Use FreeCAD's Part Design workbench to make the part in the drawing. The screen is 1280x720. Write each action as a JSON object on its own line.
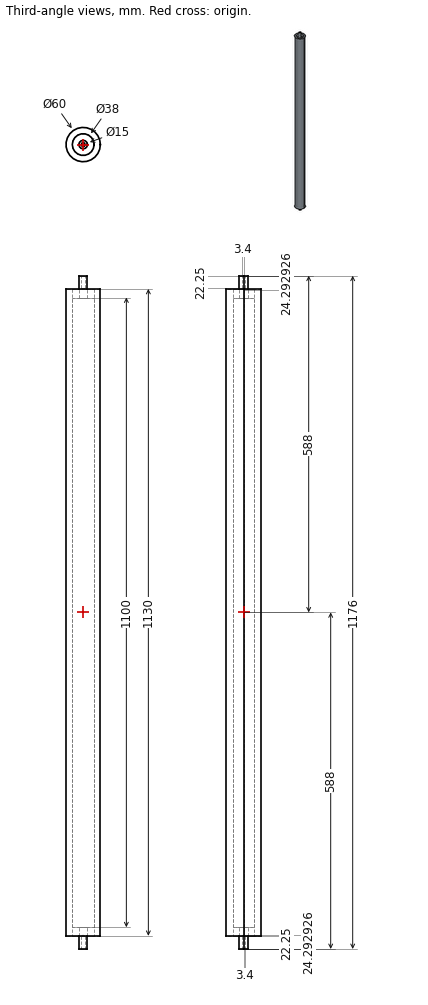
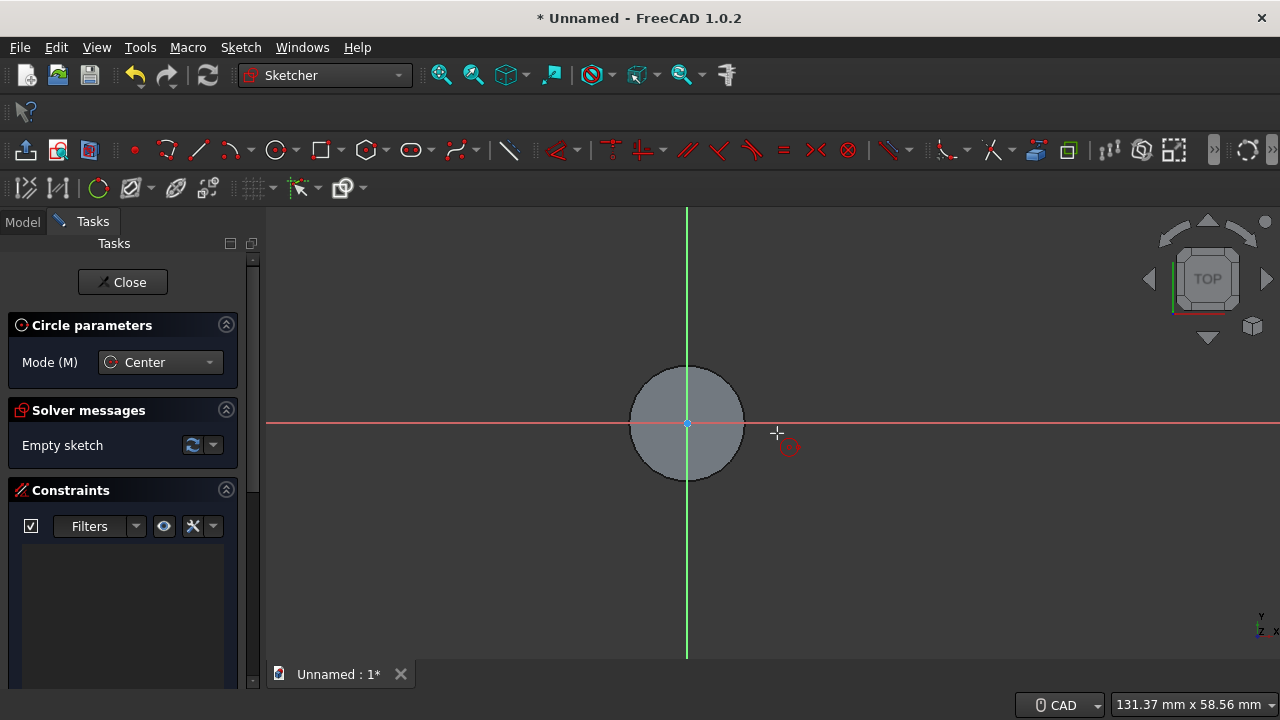
{"action": "left_click", "coordinate": [687, 423]}
{"action": "left_click", "coordinate": [791, 320]}
{"action": "key", "text": "Escape"}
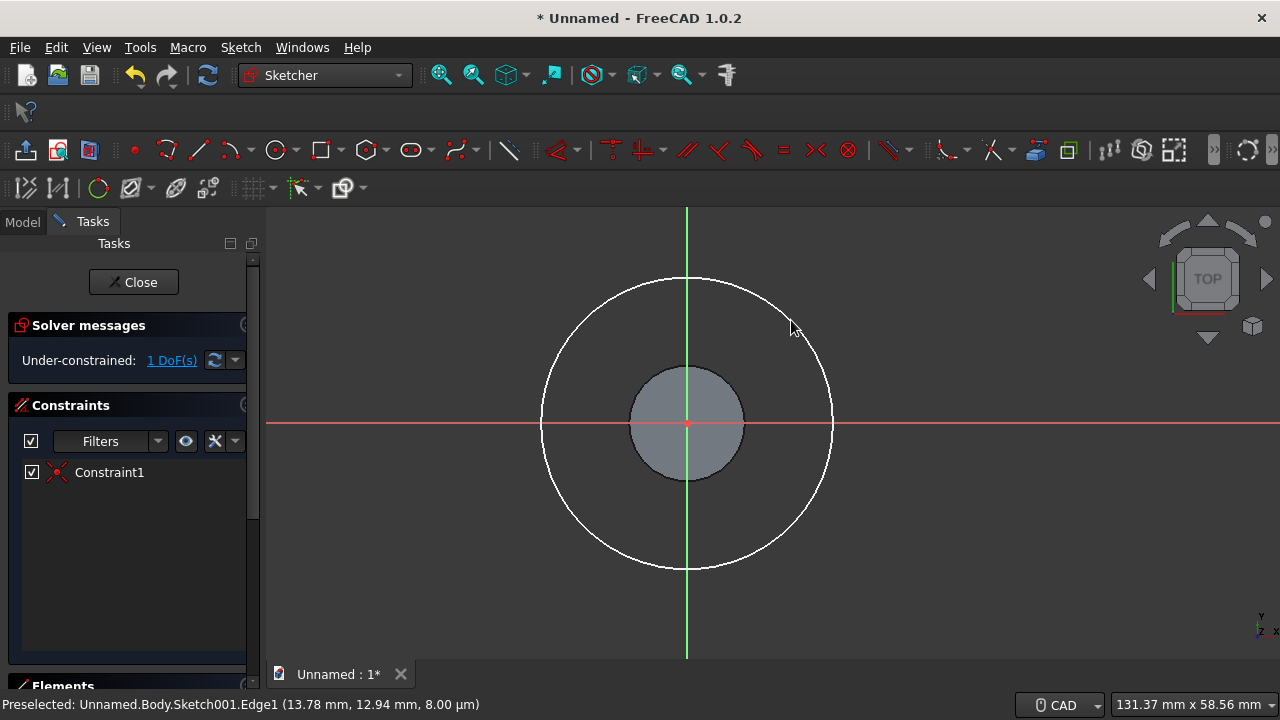
{"action": "left_click", "coordinate": [556, 150]}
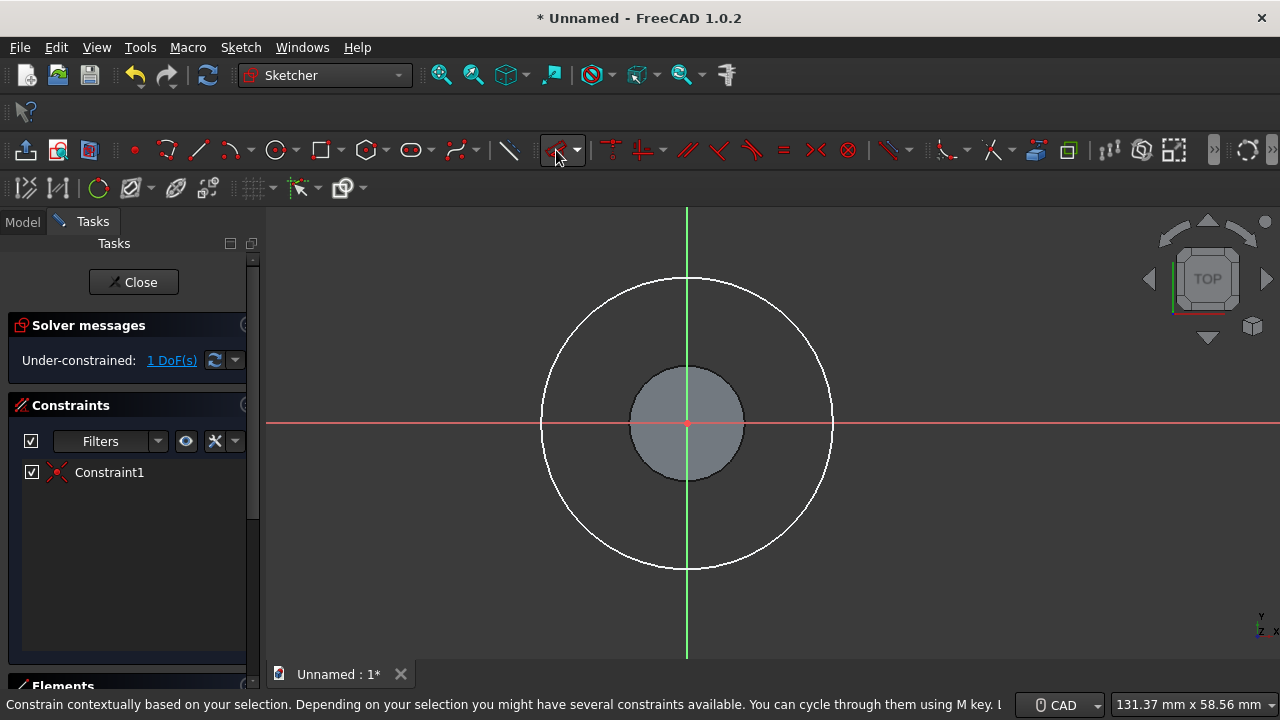
{"action": "left_click", "coordinate": [790, 320]}
{"action": "left_click", "coordinate": [813, 297]}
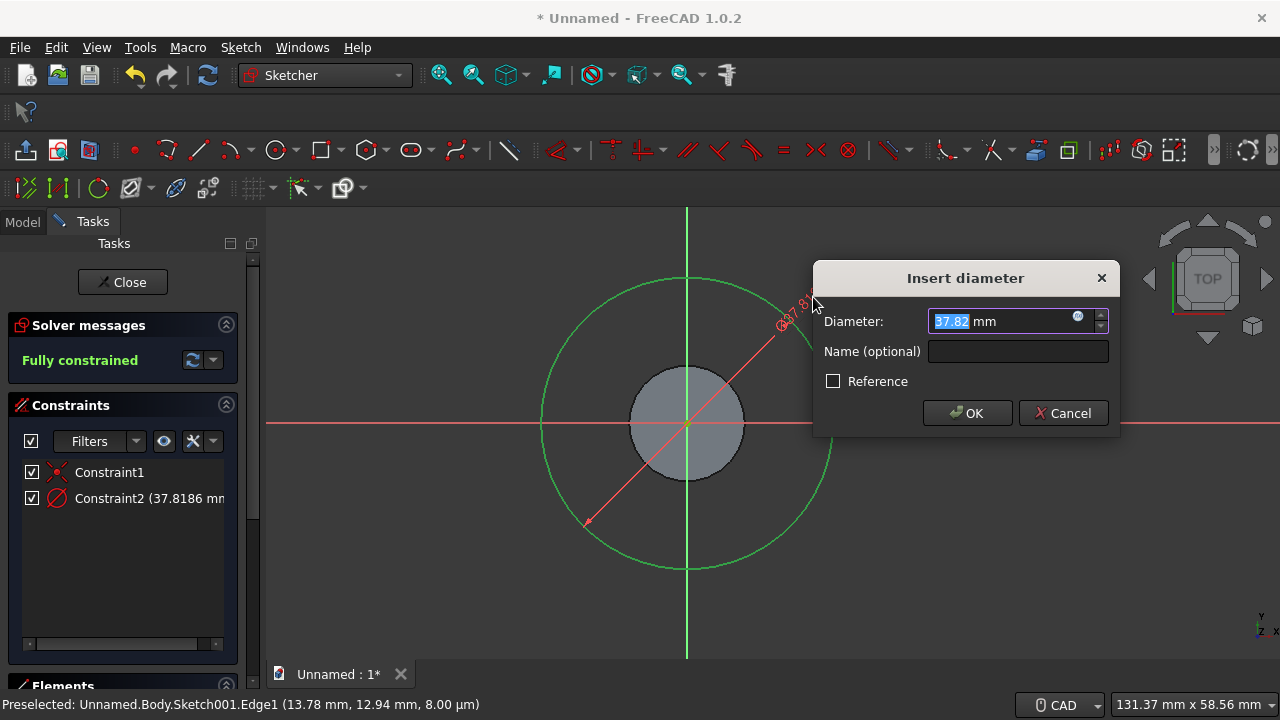
{"action": "type", "text": "38"}
{"action": "key", "text": "Return"}
{"action": "key", "text": "Escape"}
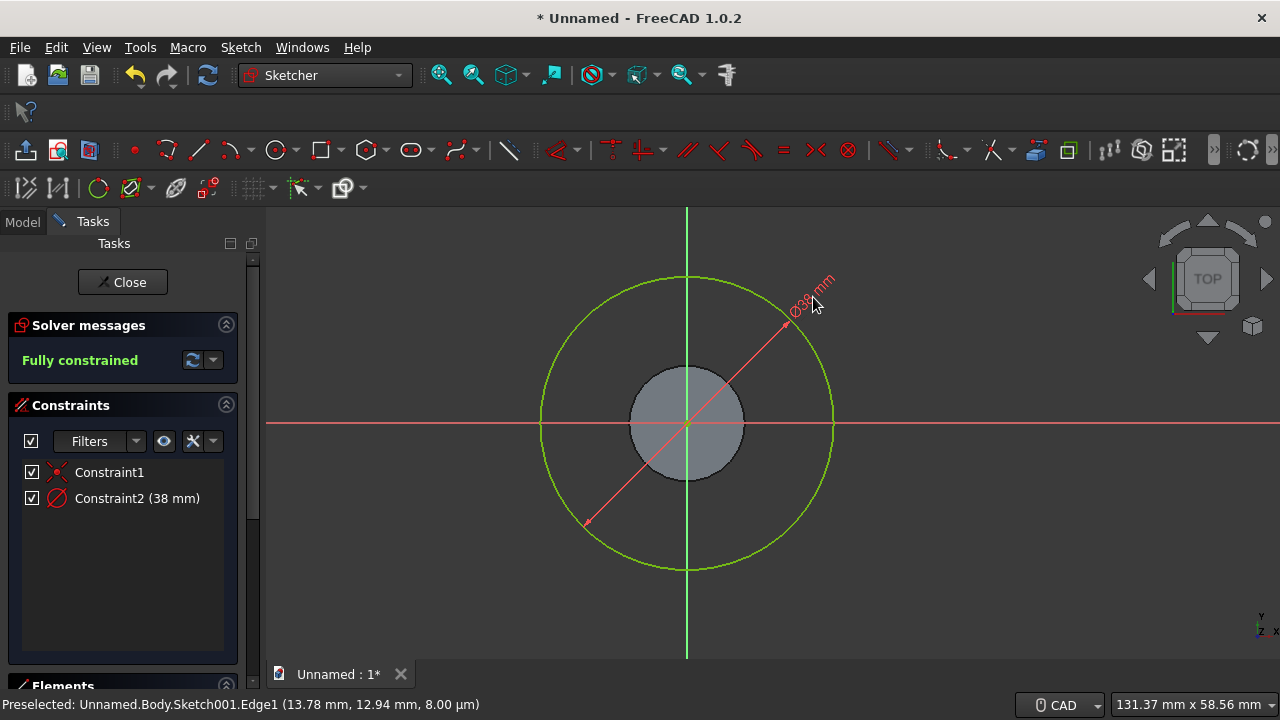
{"action": "left_click", "coordinate": [123, 282]}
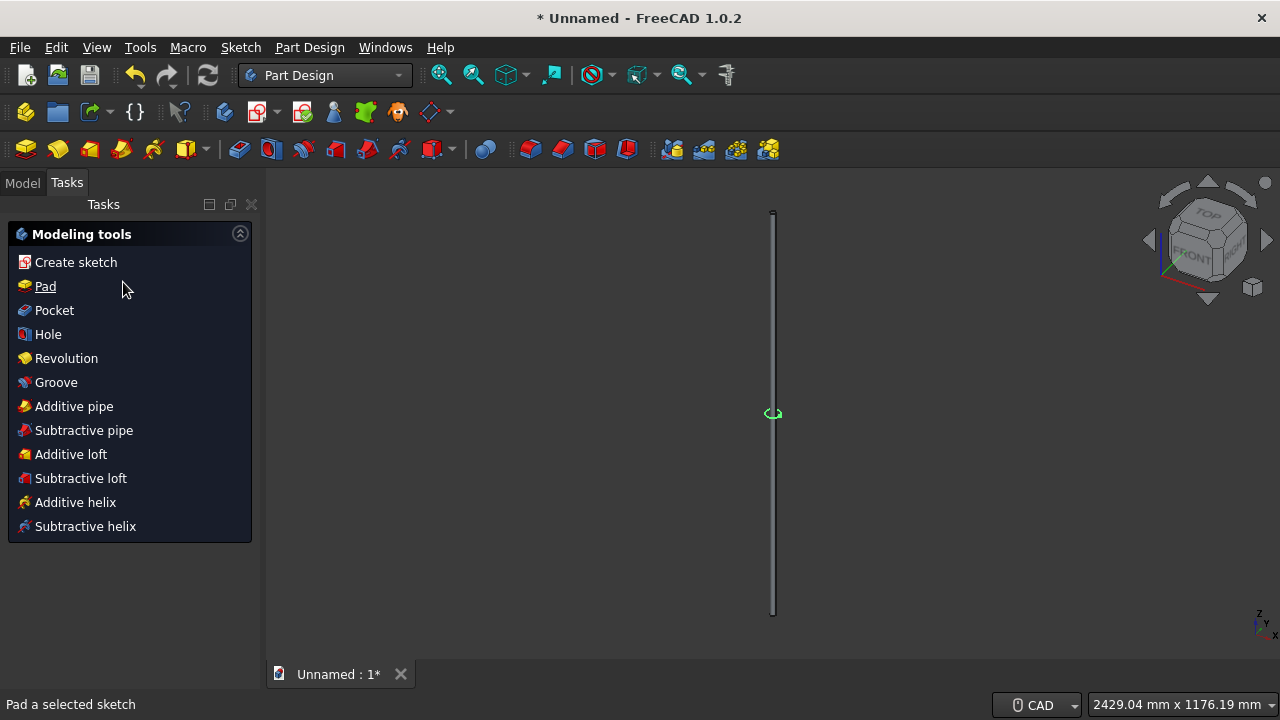
{"action": "left_click", "coordinate": [26, 150]}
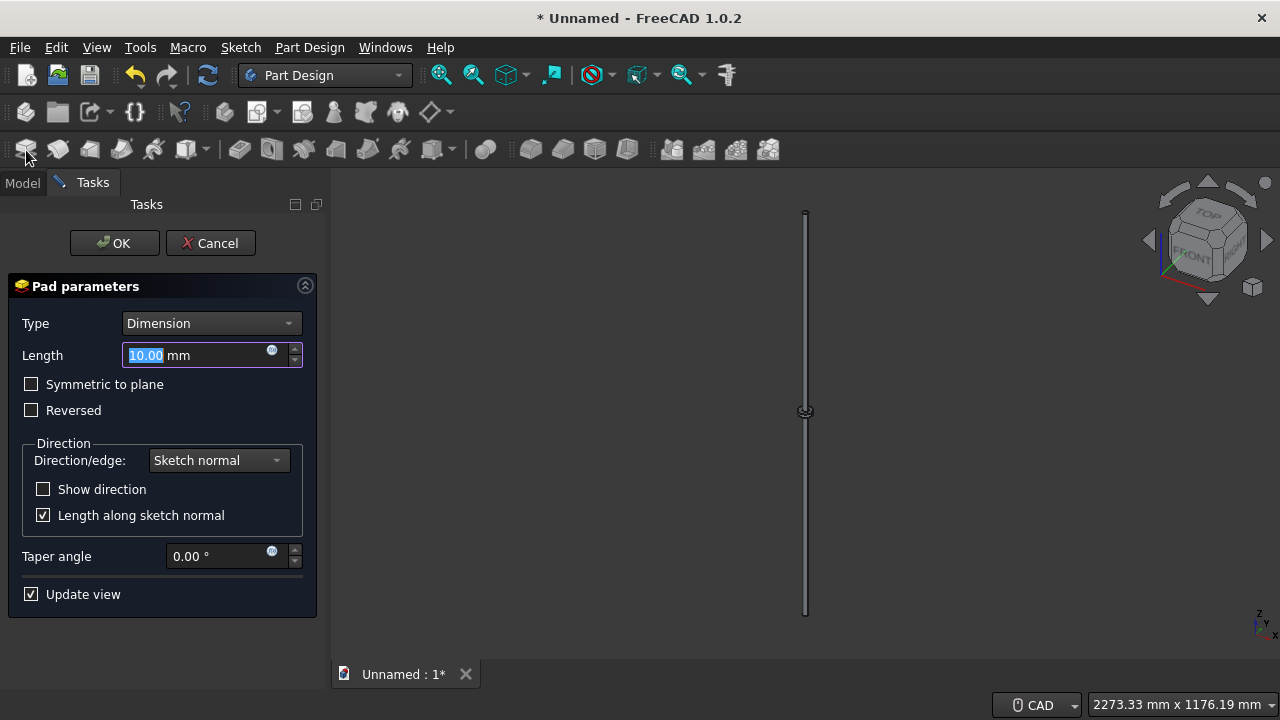
{"action": "type", "text": "1100"}
{"action": "key", "text": "Tab"}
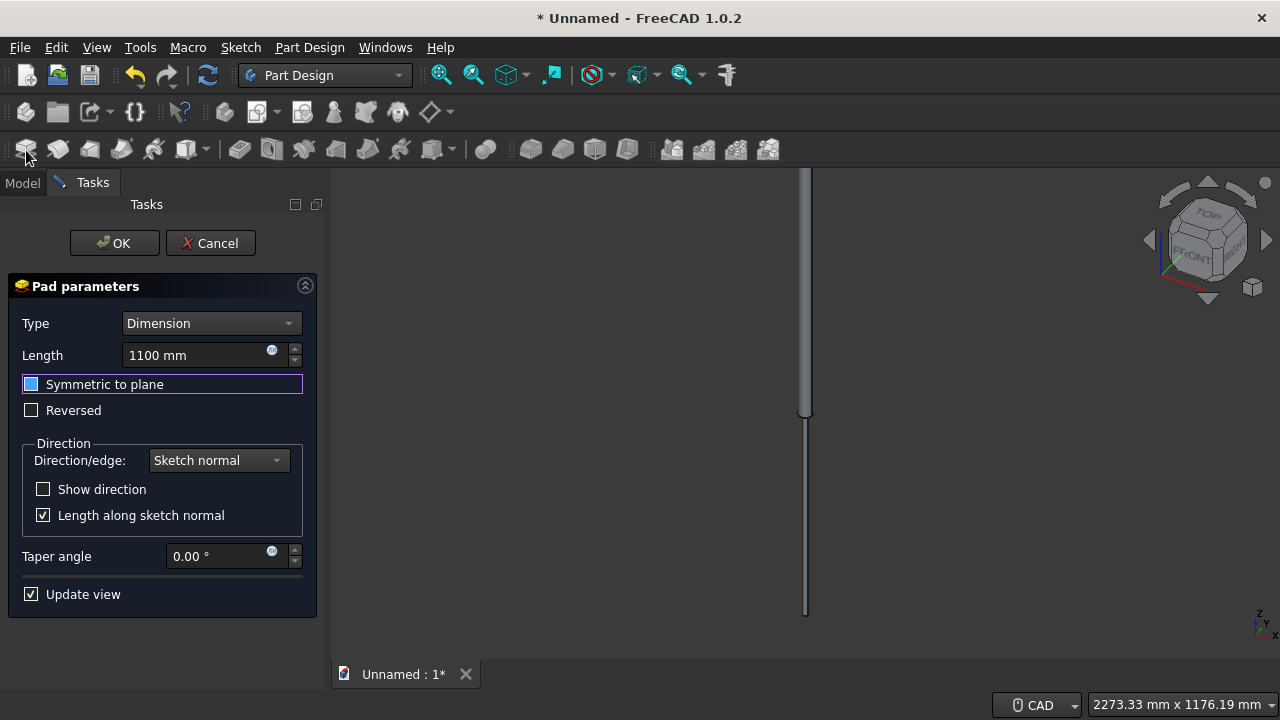
{"action": "left_click", "coordinate": [30, 384]}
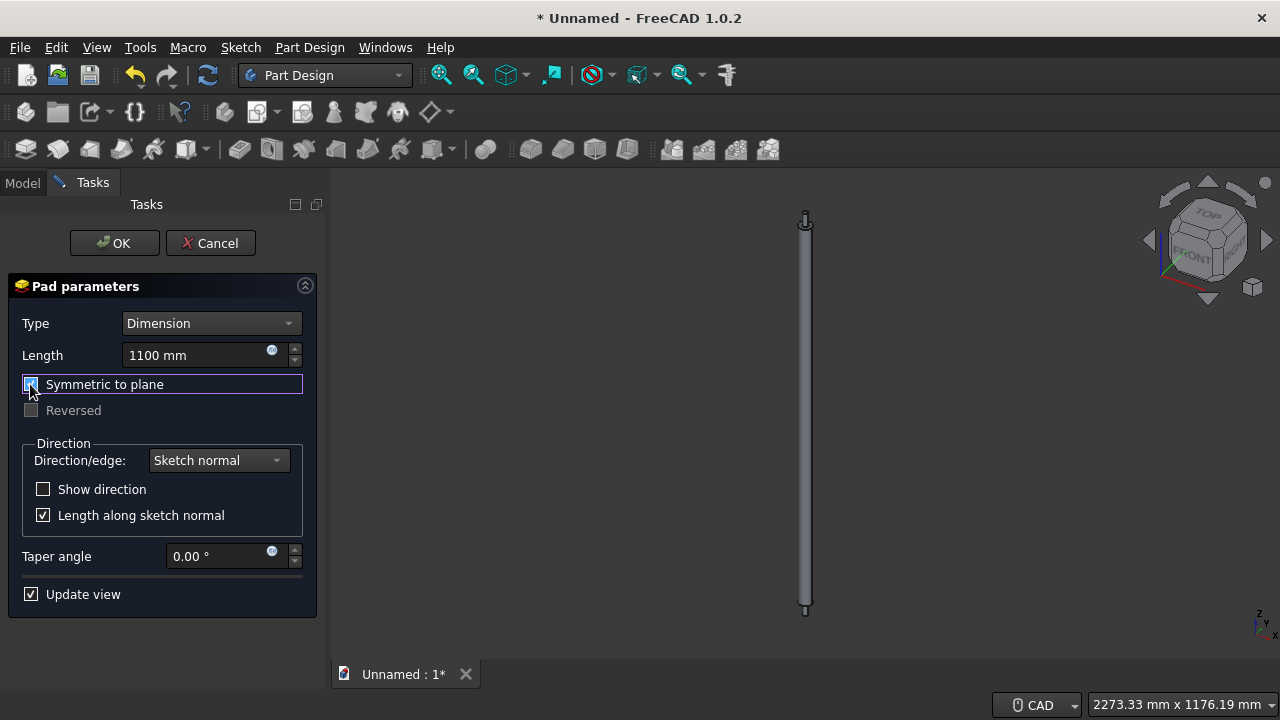
{"action": "left_click", "coordinate": [115, 243]}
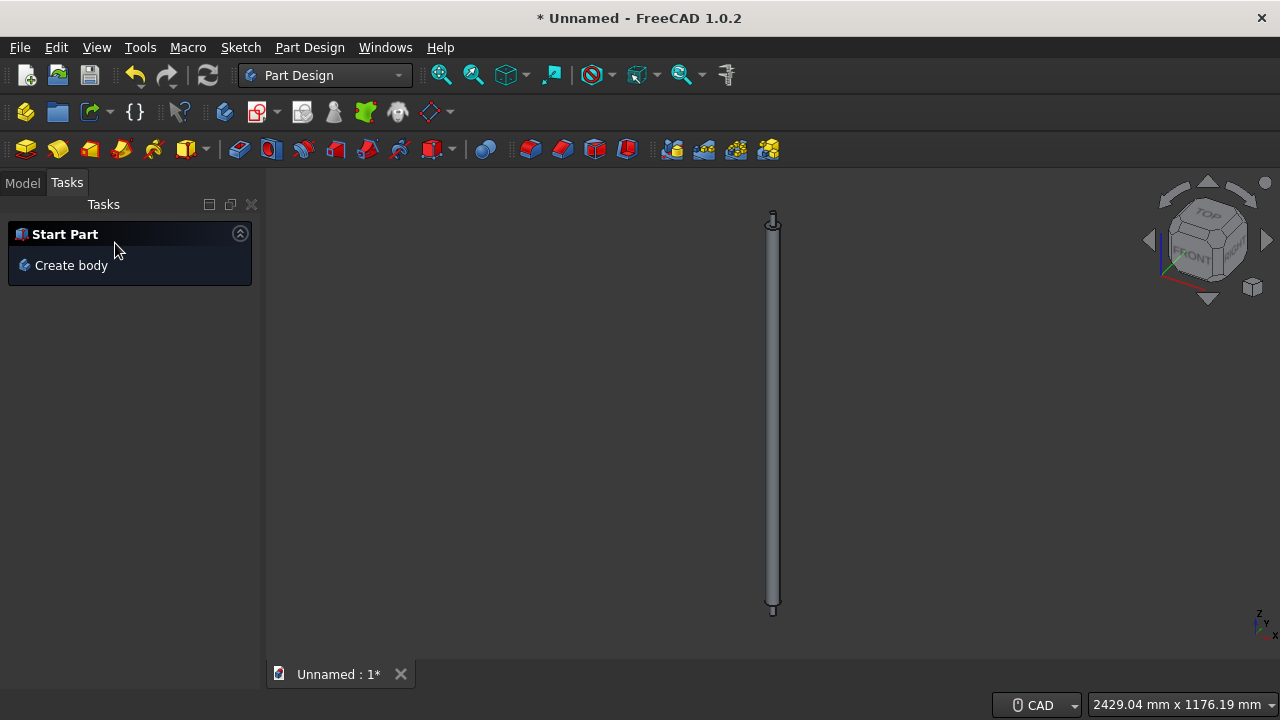
{"action": "left_click", "coordinate": [258, 112]}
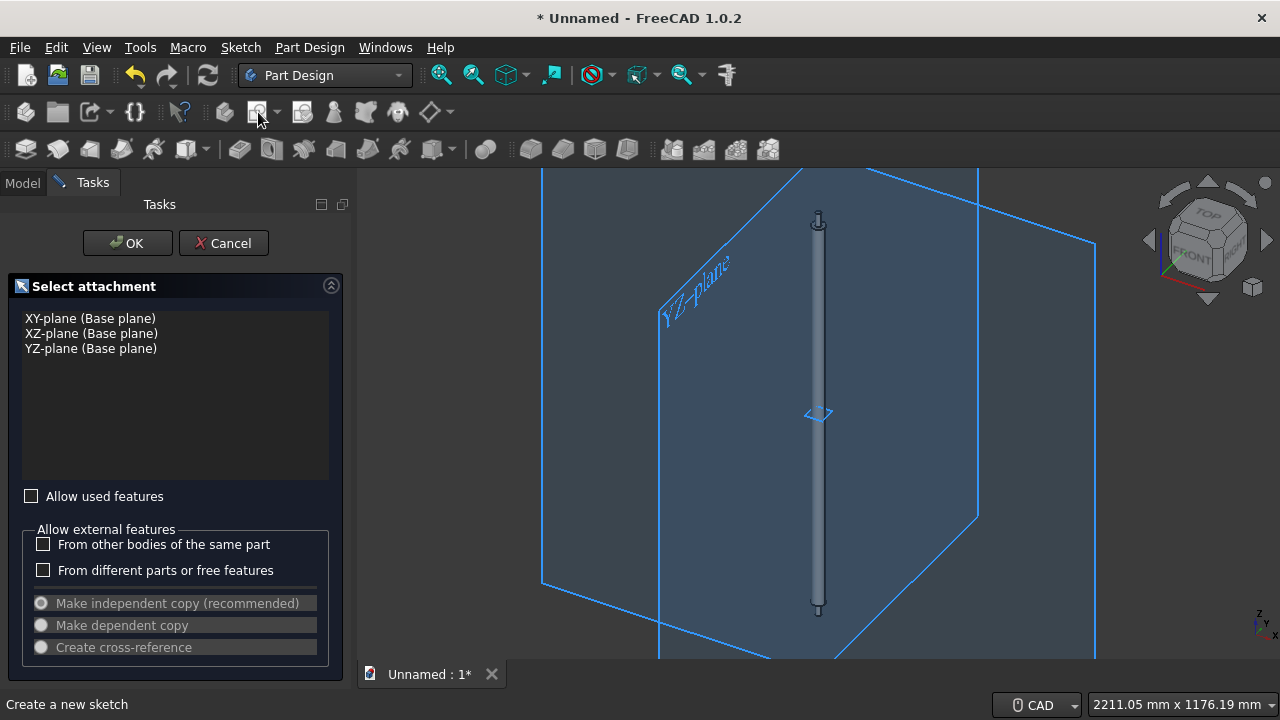
{"action": "left_click", "coordinate": [82, 348]}